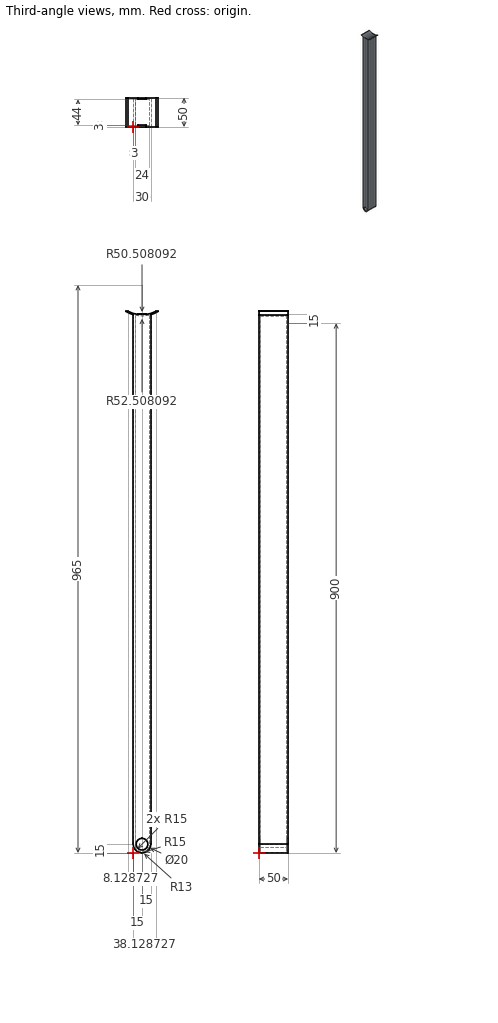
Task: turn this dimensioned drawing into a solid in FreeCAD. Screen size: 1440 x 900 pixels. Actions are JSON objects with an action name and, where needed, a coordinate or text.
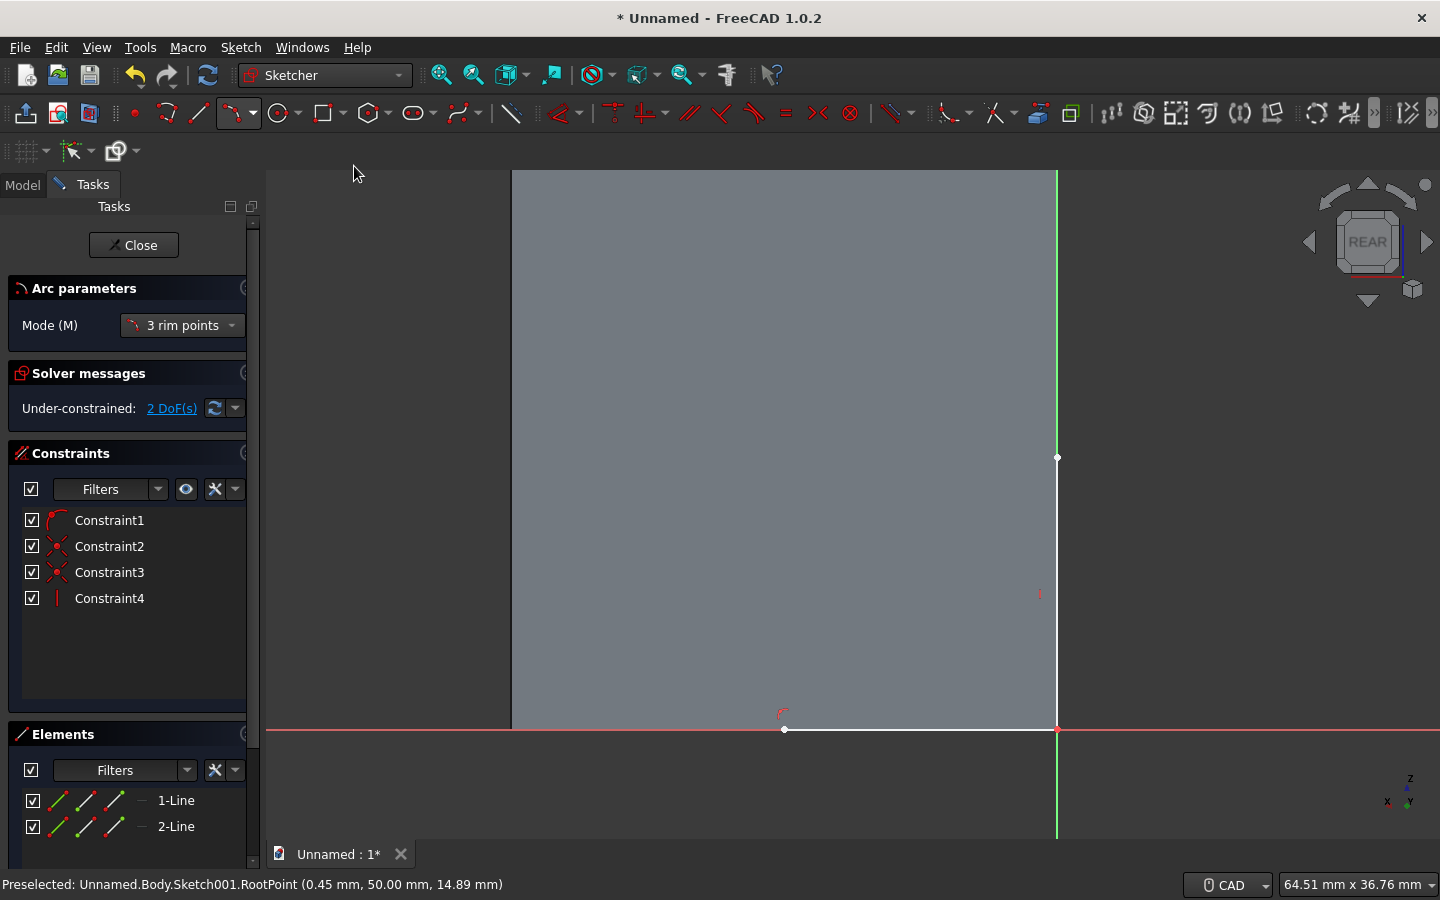
{"action": "left_click", "coordinate": [1048, 457]}
{"action": "left_click", "coordinate": [784, 730]}
{"action": "left_click", "coordinate": [977, 650]}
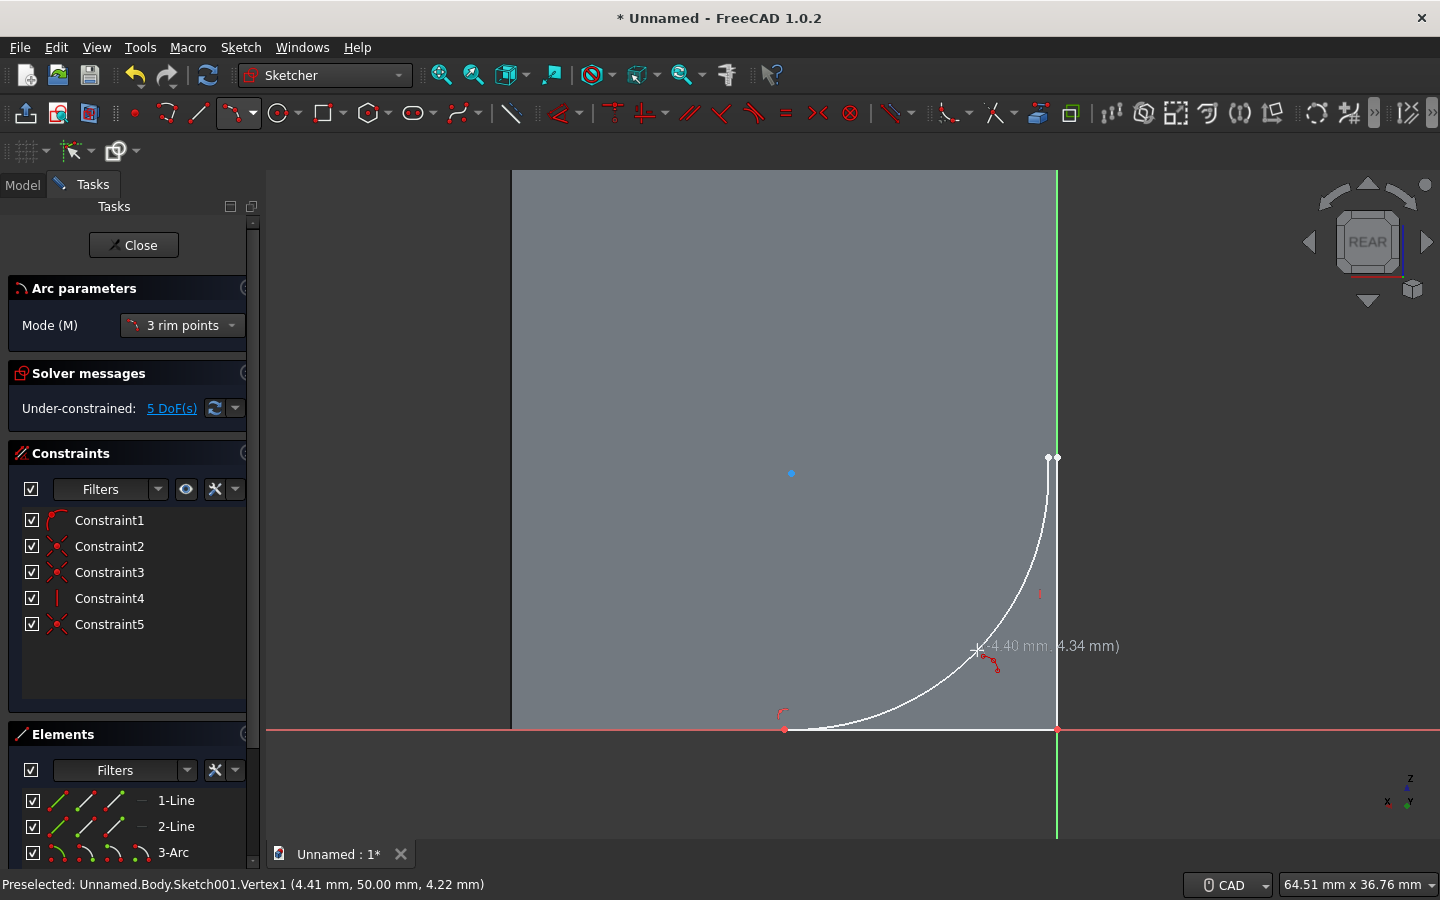
{"action": "left_click", "coordinate": [168, 114]}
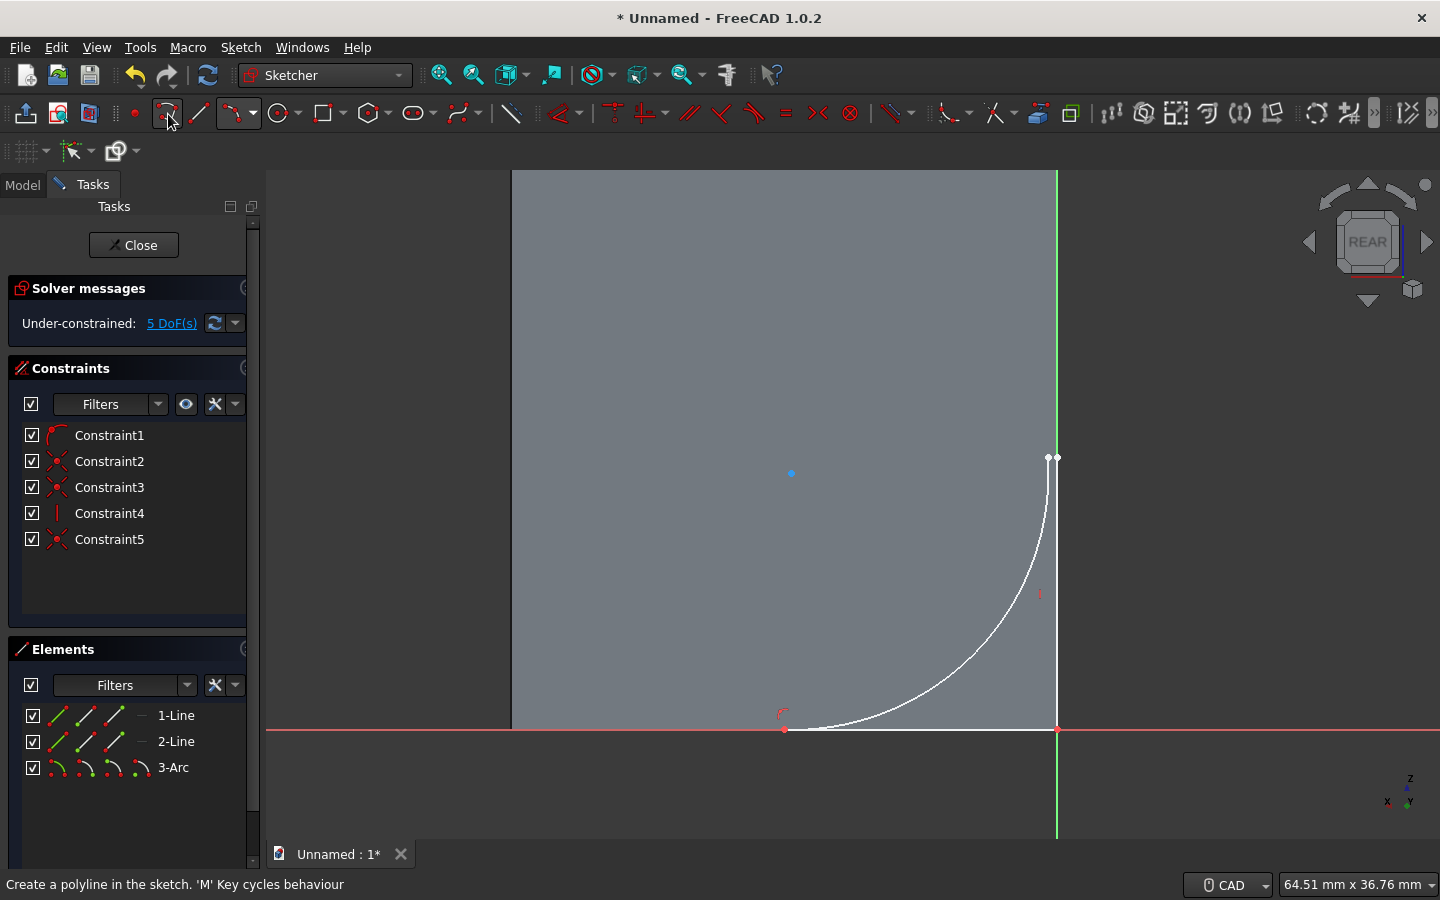
{"action": "left_click", "coordinate": [511, 457]}
{"action": "left_click", "coordinate": [511, 721]}
{"action": "left_click", "coordinate": [784, 730]}
{"action": "right_click", "coordinate": [511, 721]}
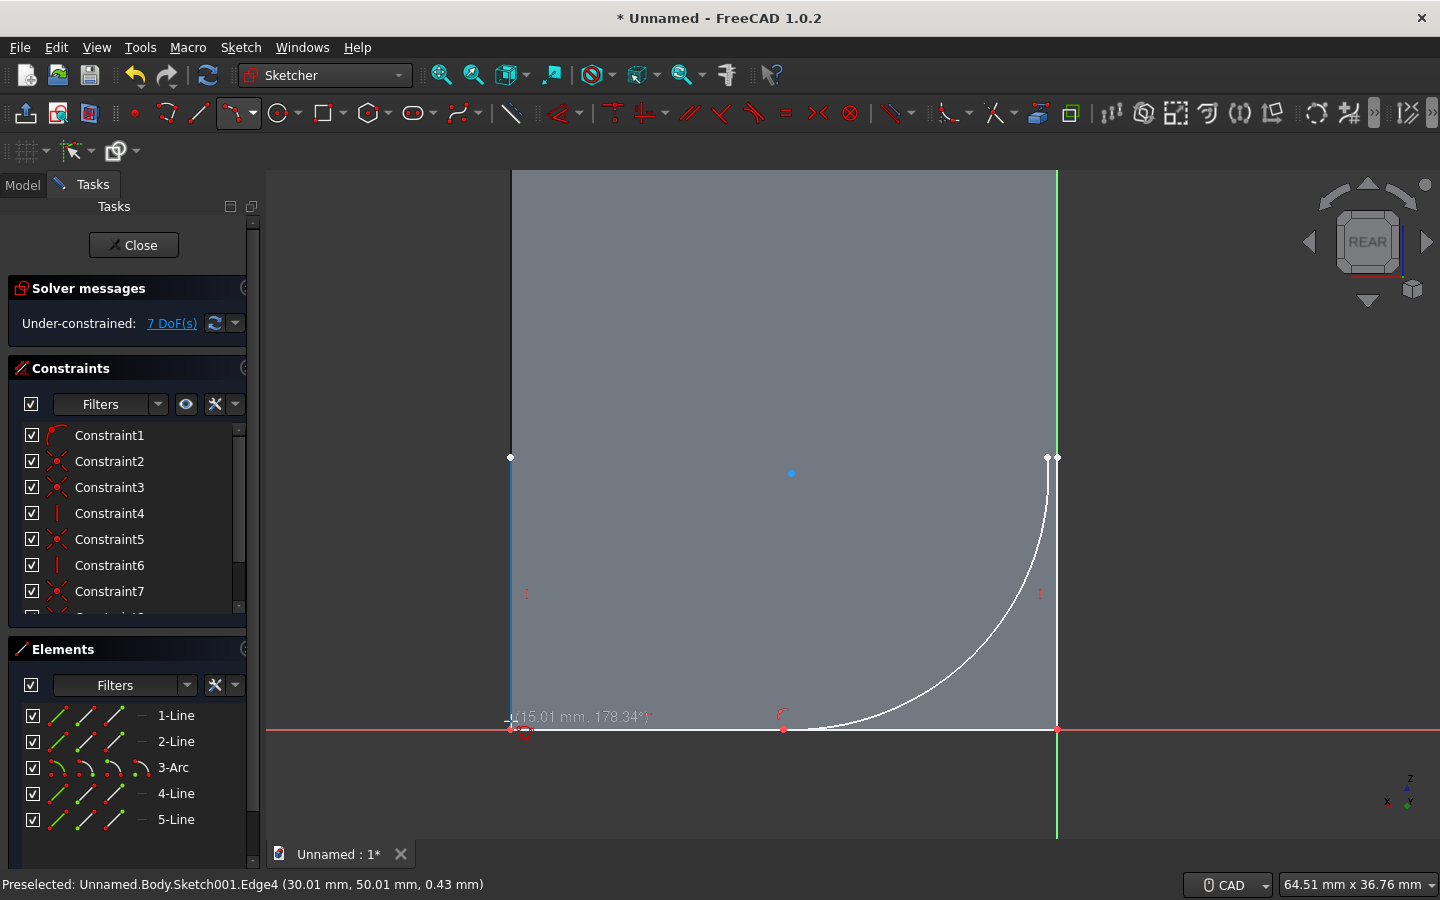
{"action": "left_click", "coordinate": [232, 114]}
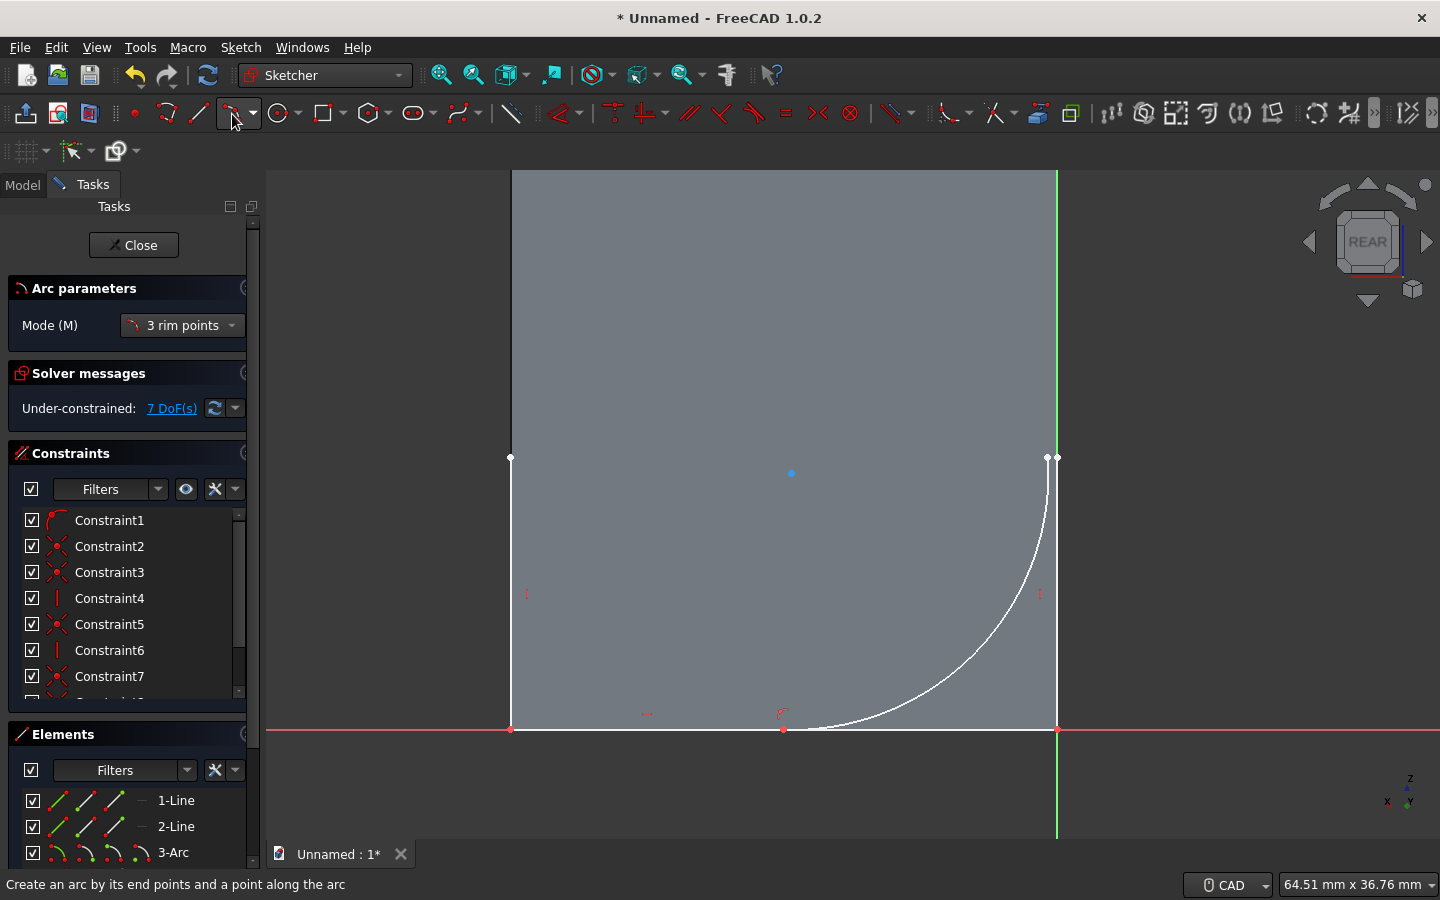
{"action": "left_click", "coordinate": [784, 730]}
{"action": "left_click", "coordinate": [511, 458]}
{"action": "left_click", "coordinate": [591, 650]}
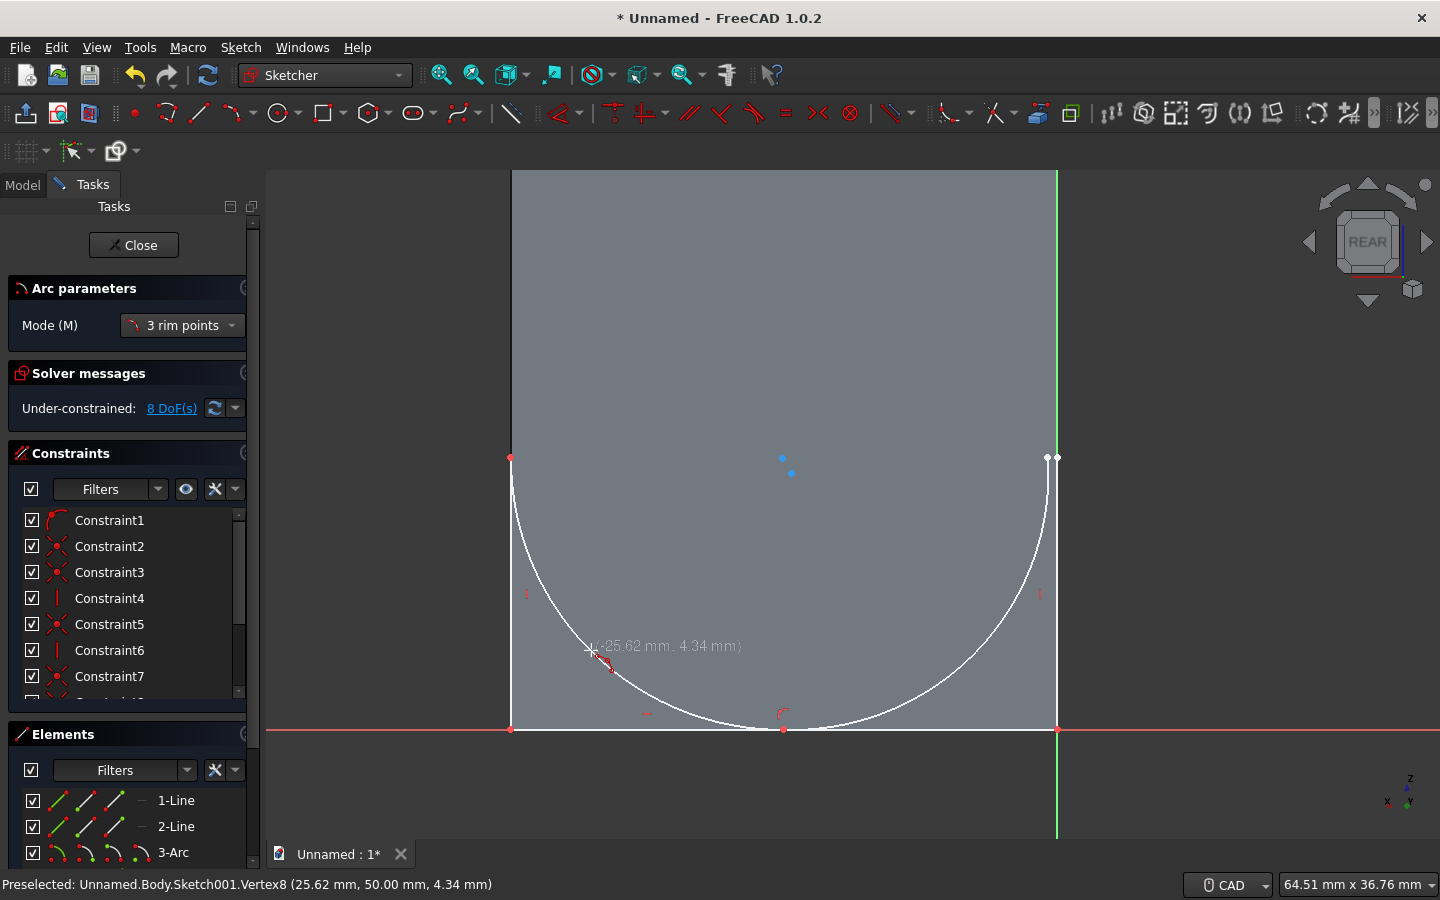
{"action": "left_click", "coordinate": [278, 114]}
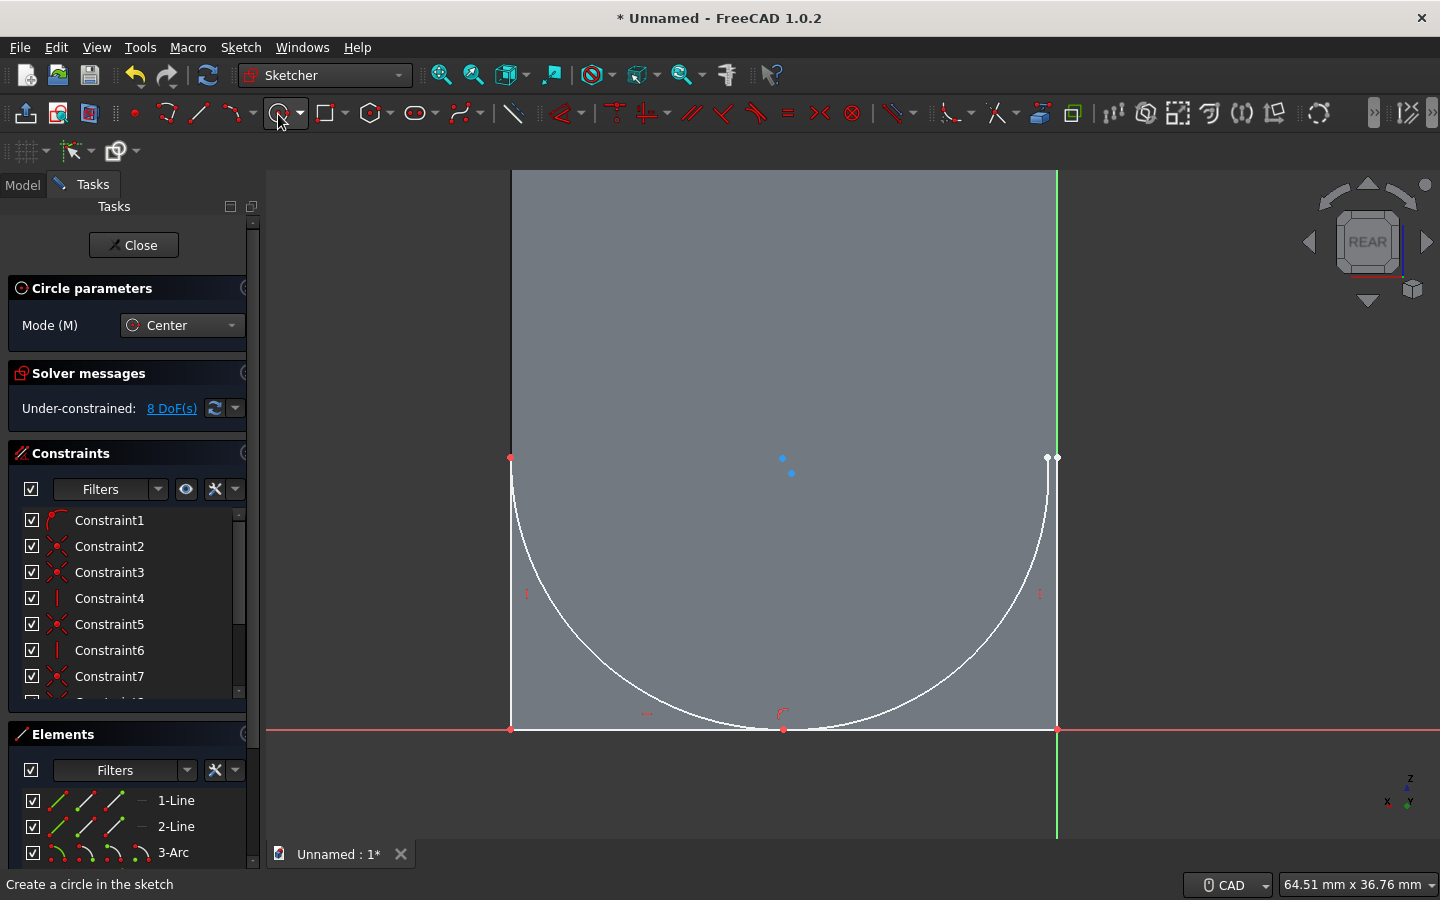
{"action": "left_click", "coordinate": [784, 457]}
{"action": "left_click", "coordinate": [913, 328]}
{"action": "key", "text": "Escape"}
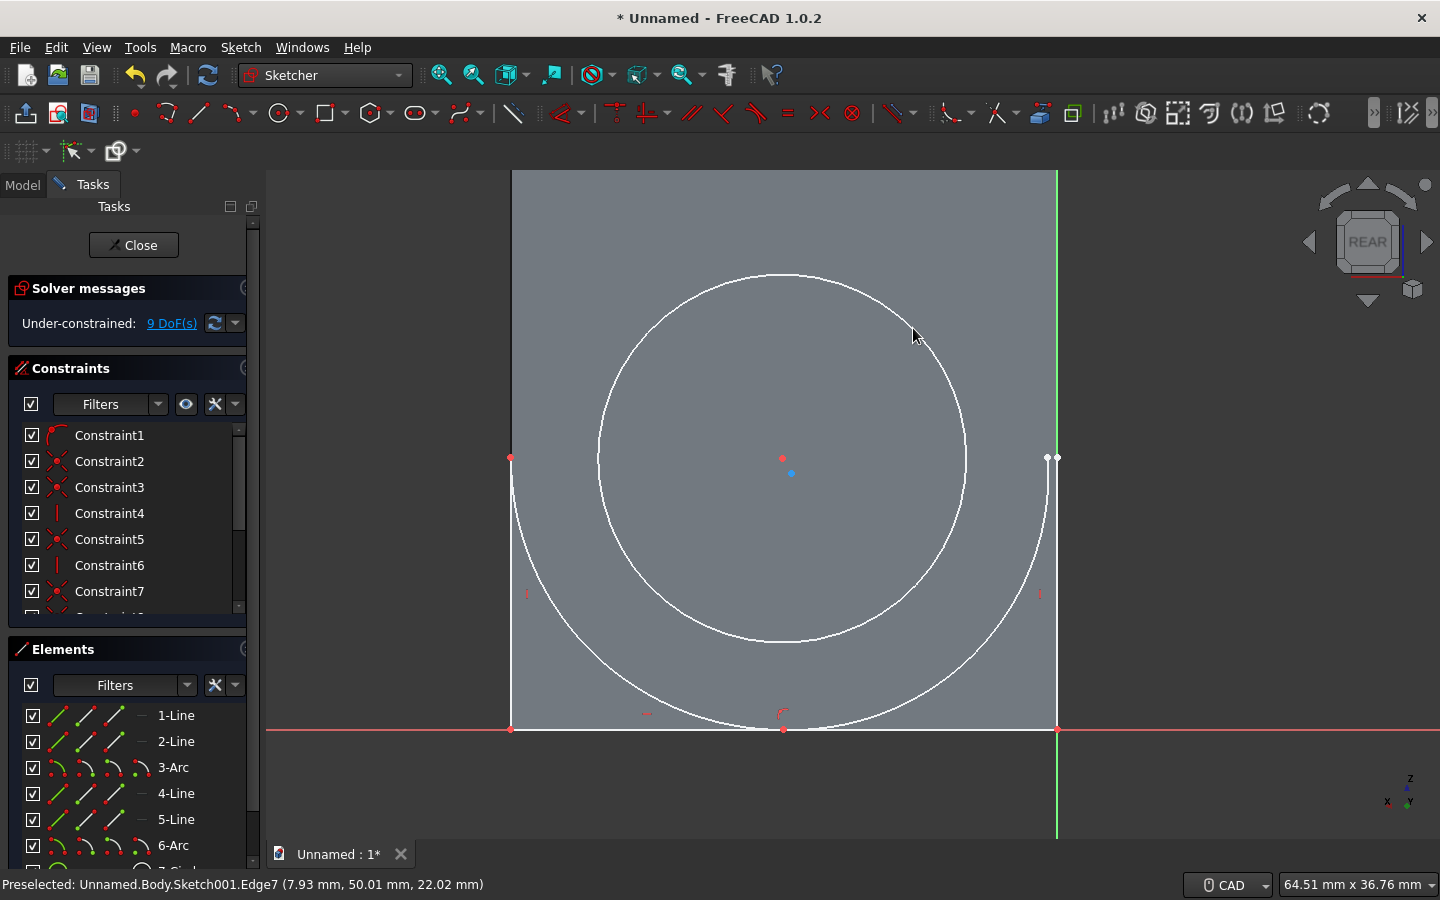
{"action": "scroll", "coordinate": [866, 730], "scroll_direction": "up", "scroll_amount": 2}